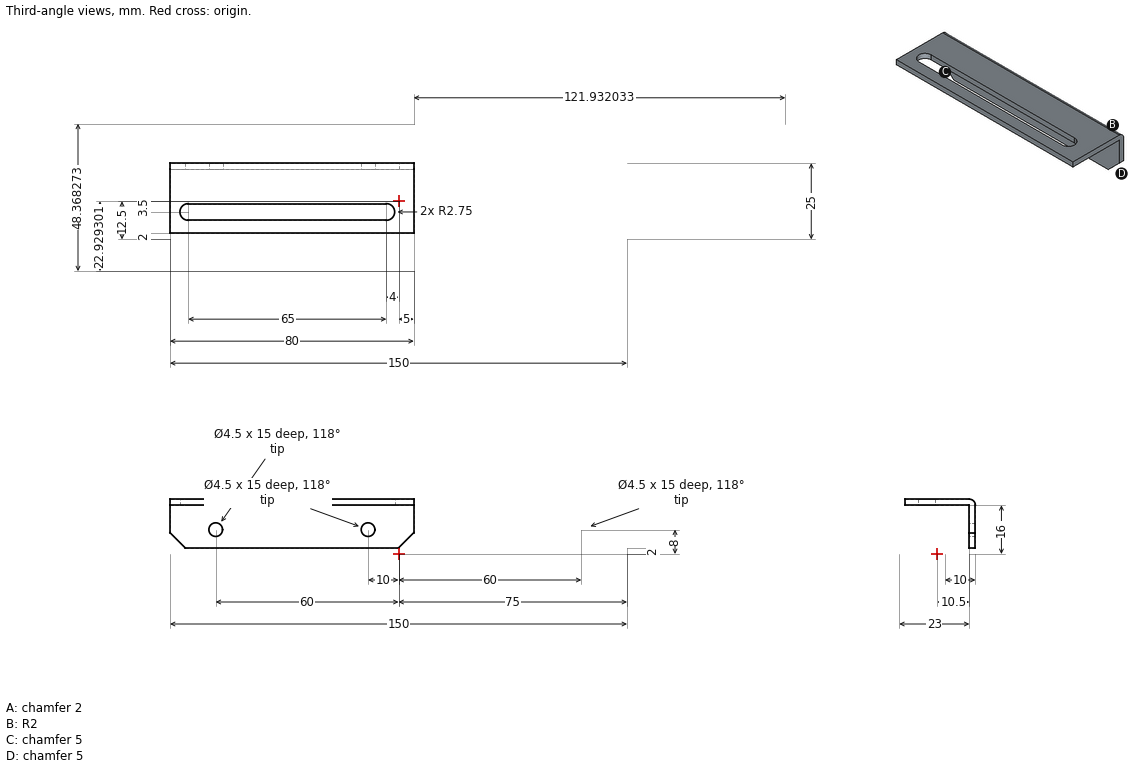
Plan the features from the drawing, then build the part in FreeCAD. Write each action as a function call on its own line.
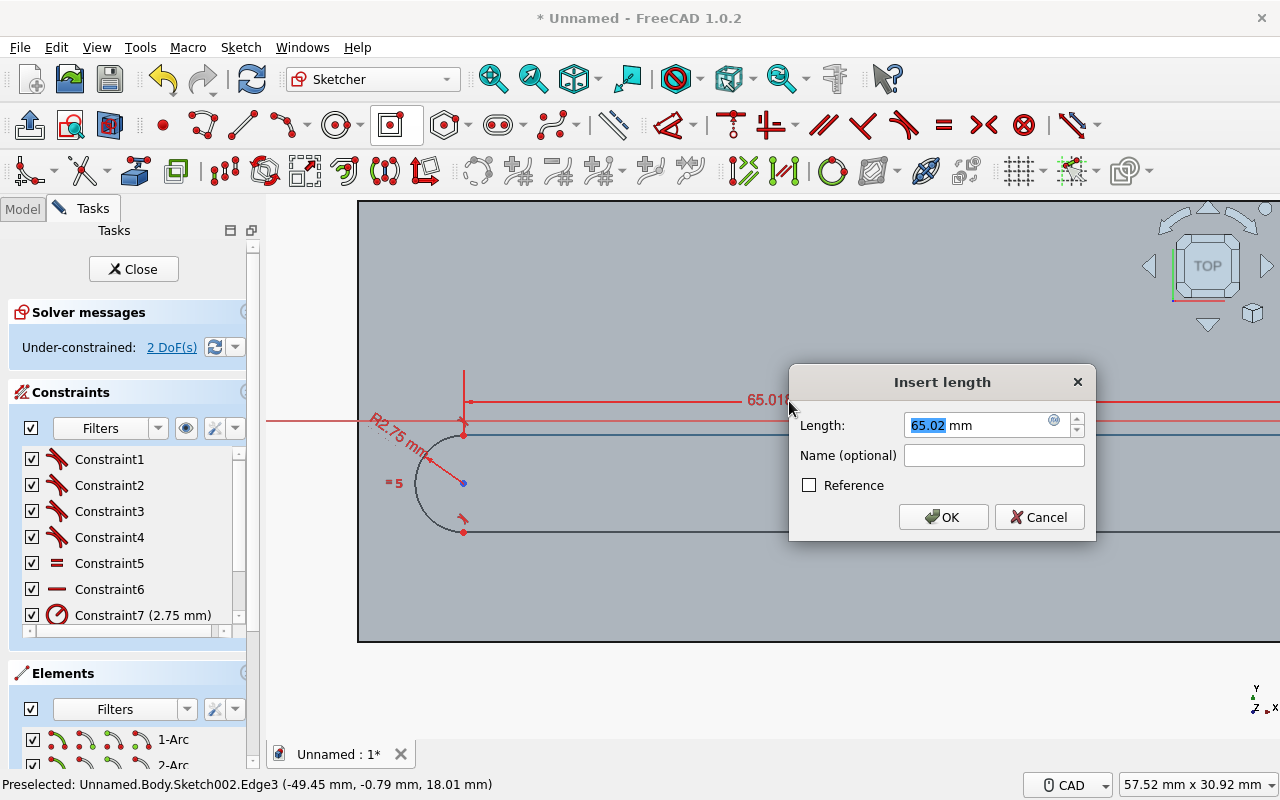
text(65)
key(Return)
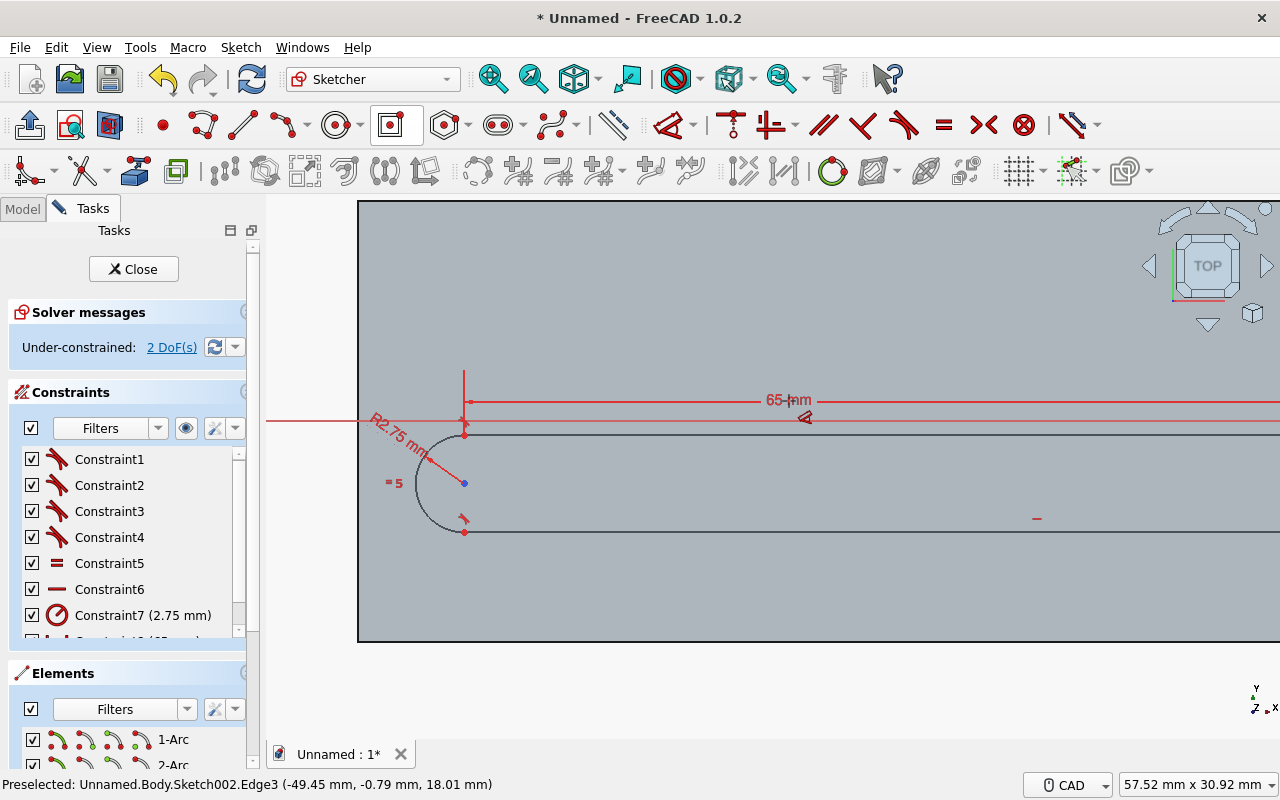
scroll(425, 458, down, 4)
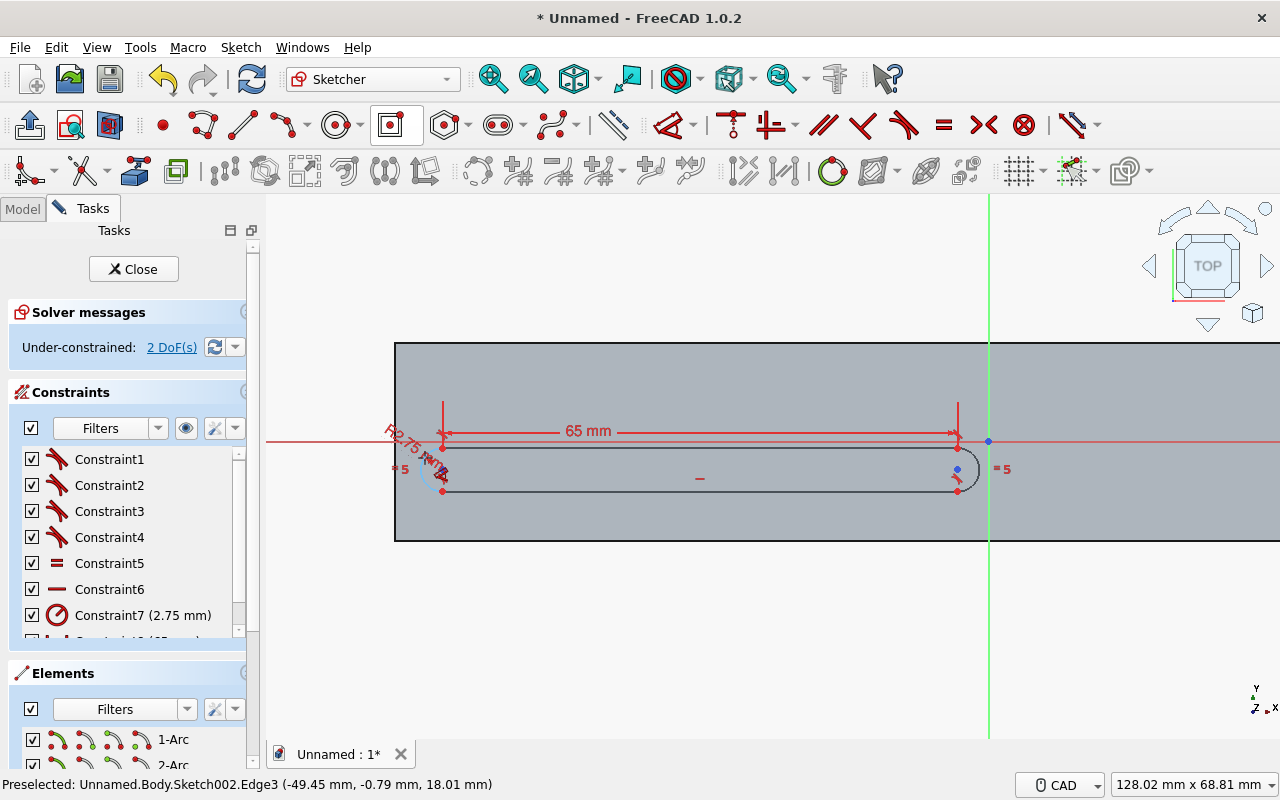
scroll(958, 492, up, 2)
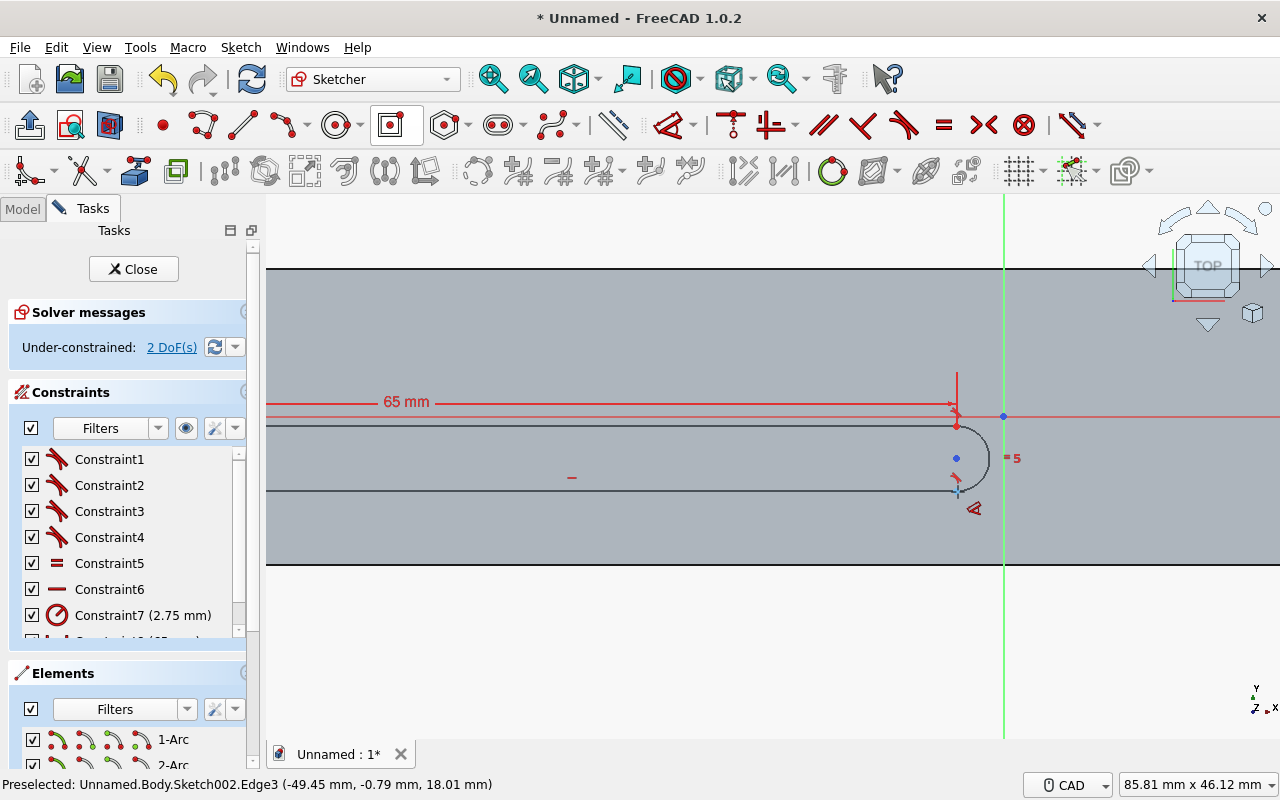
click(957, 491)
click(980, 525)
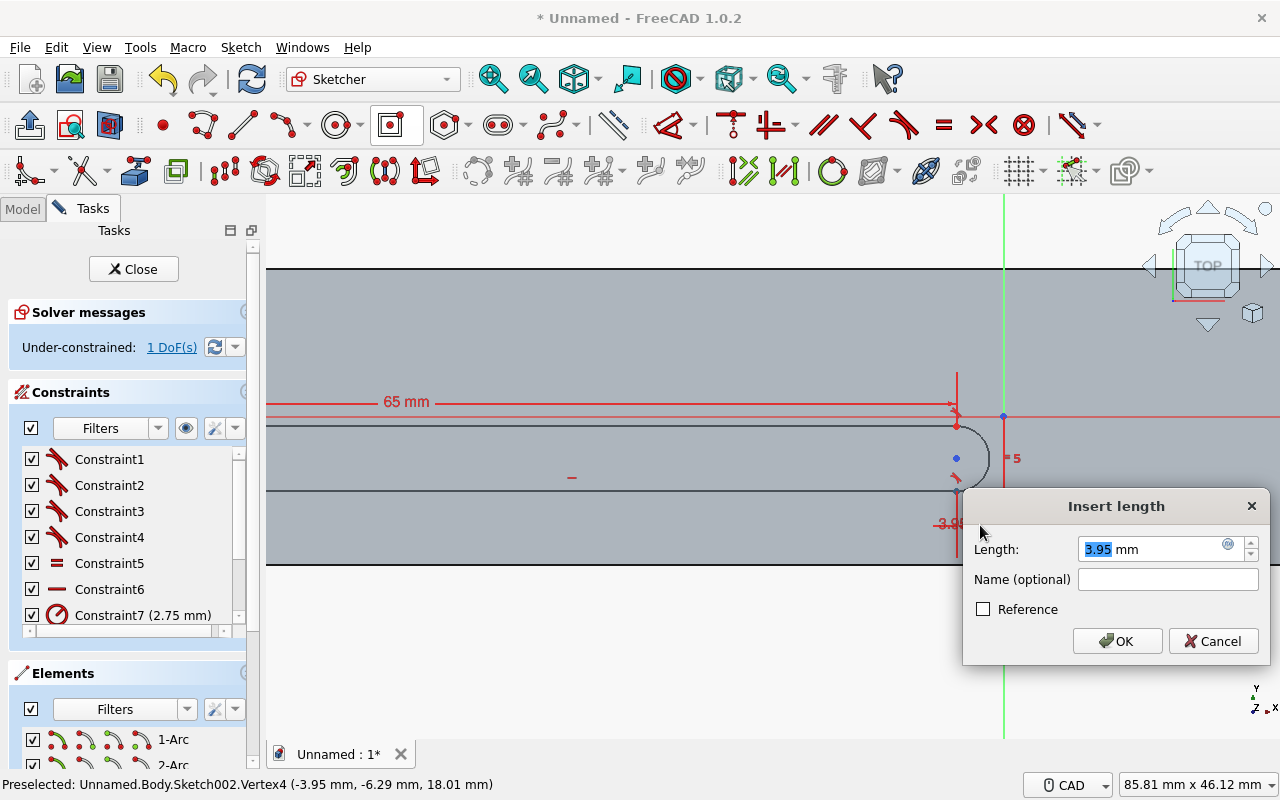
text(4)
key(Return)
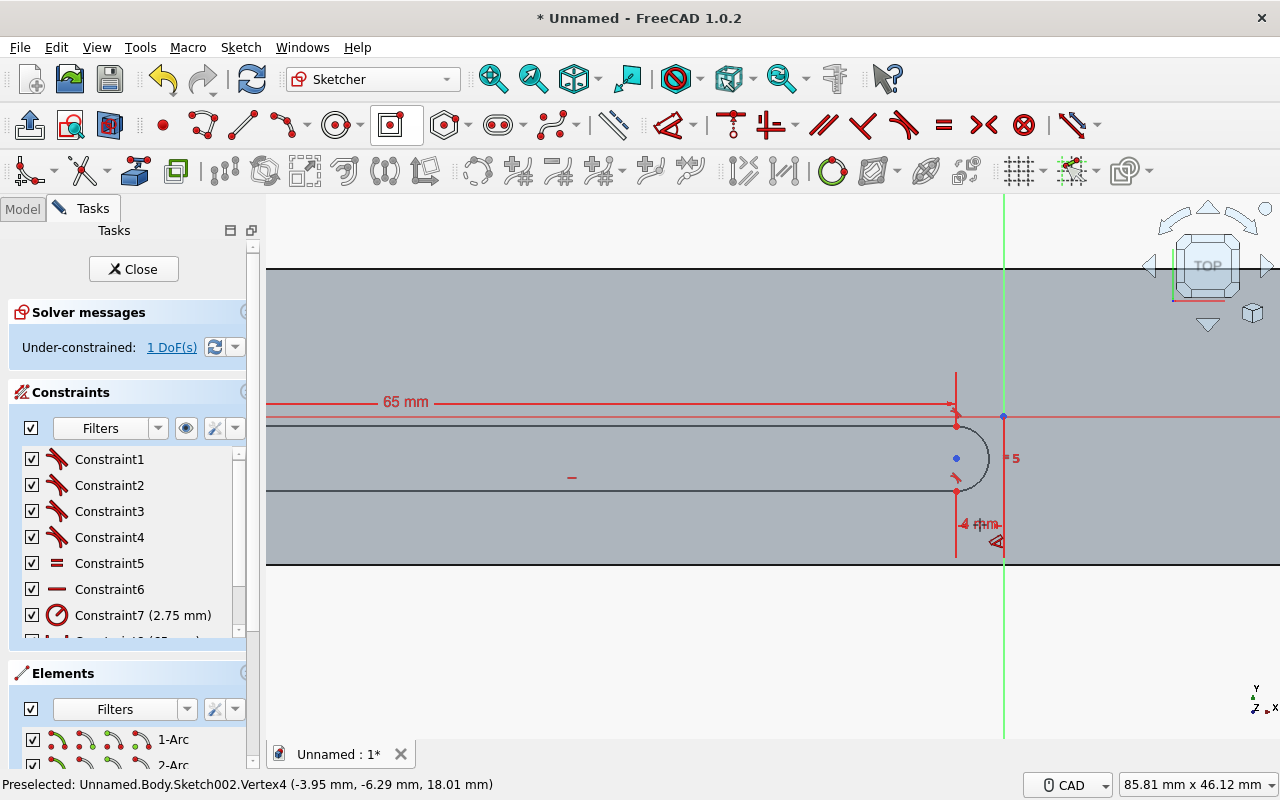
scroll(958, 492, down, 2)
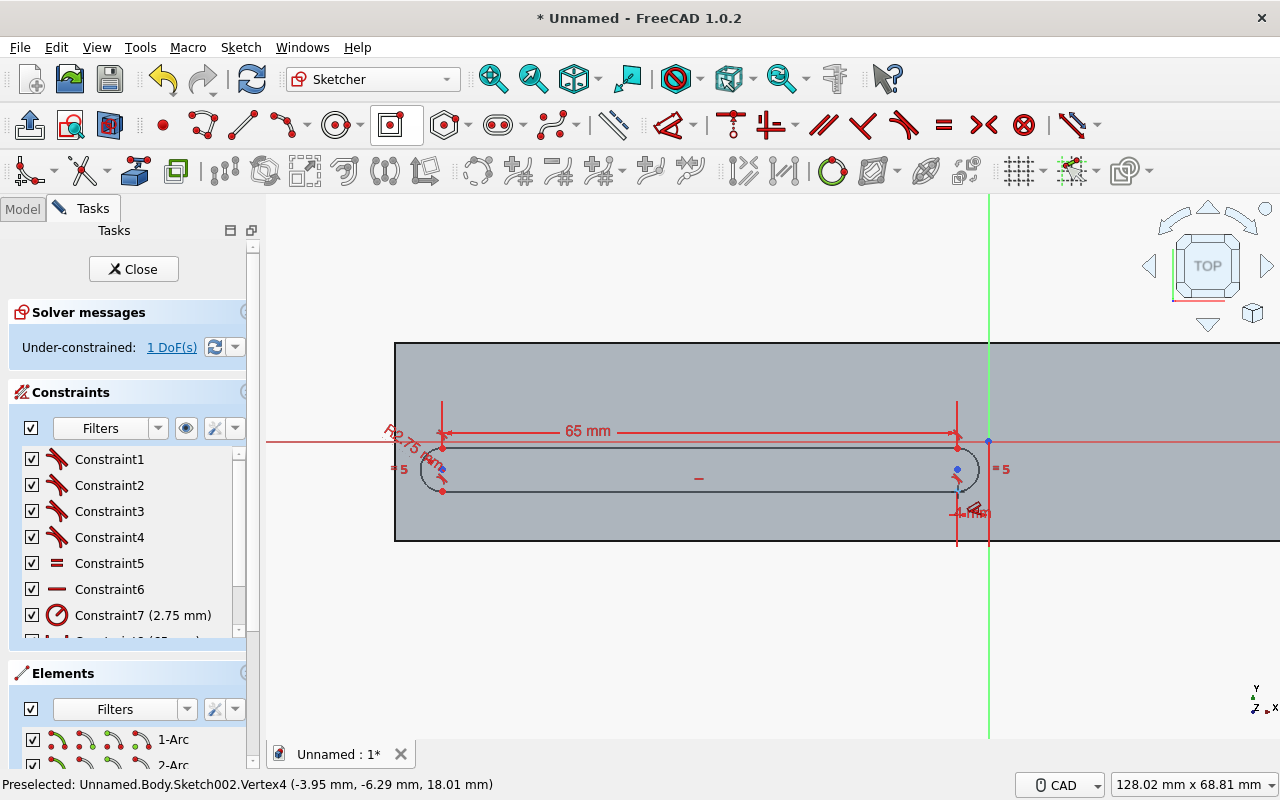
scroll(442, 470, up, 2)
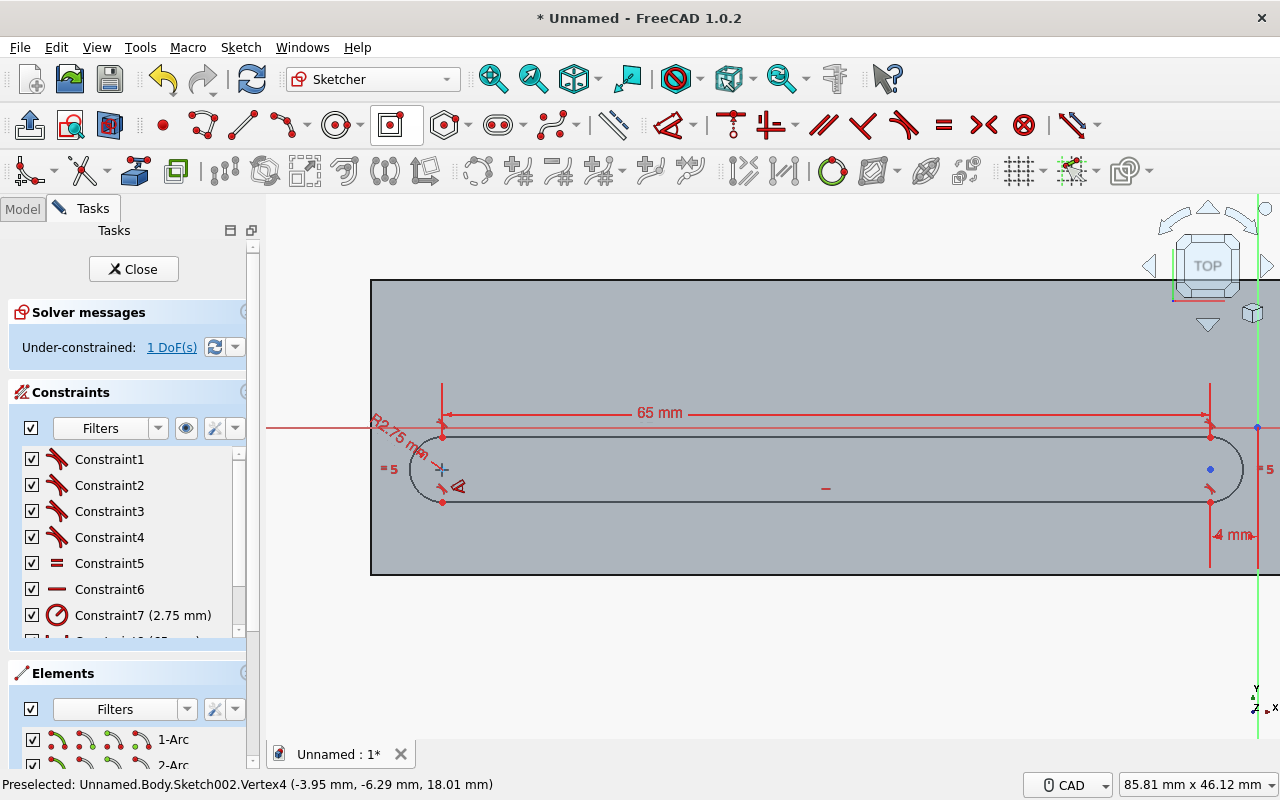
click(442, 470)
click(384, 463)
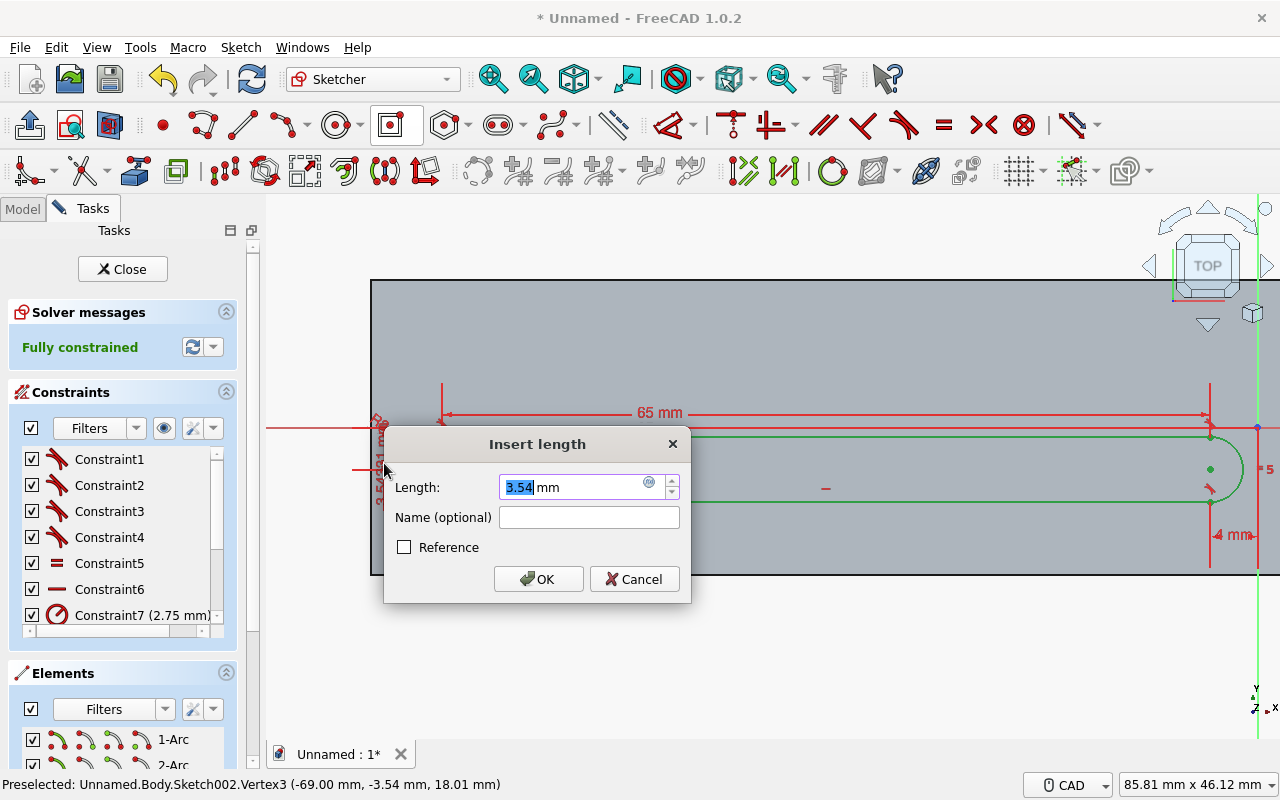
text(3.5)
key(Return)
key(Escape)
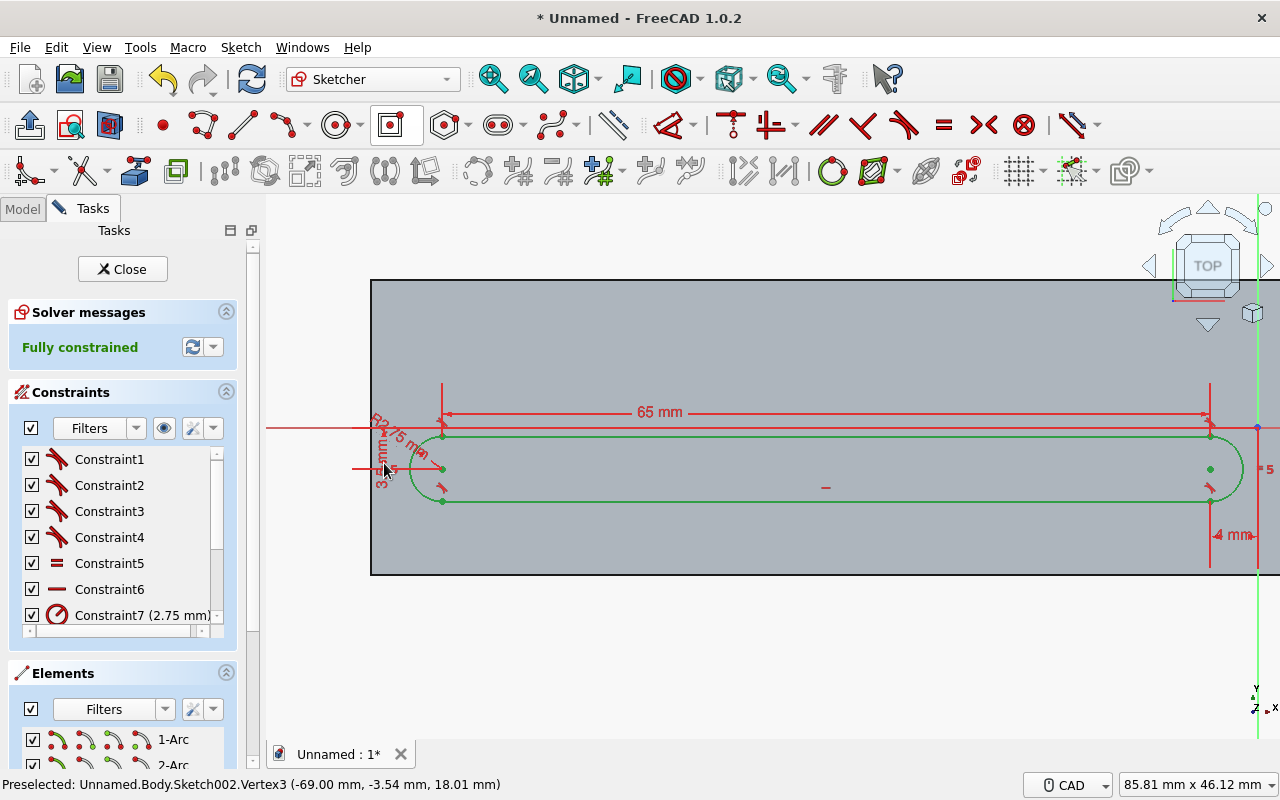
click(123, 269)